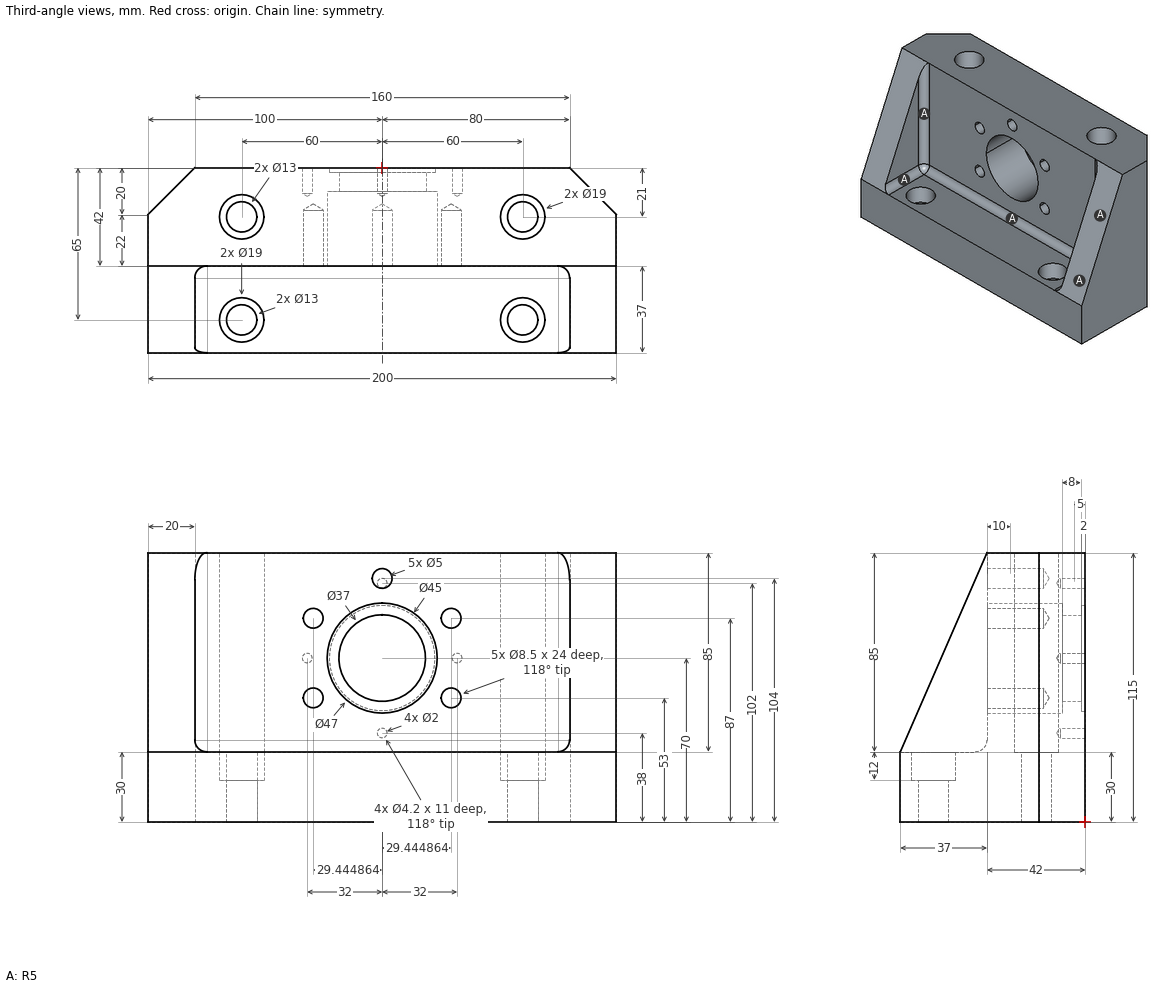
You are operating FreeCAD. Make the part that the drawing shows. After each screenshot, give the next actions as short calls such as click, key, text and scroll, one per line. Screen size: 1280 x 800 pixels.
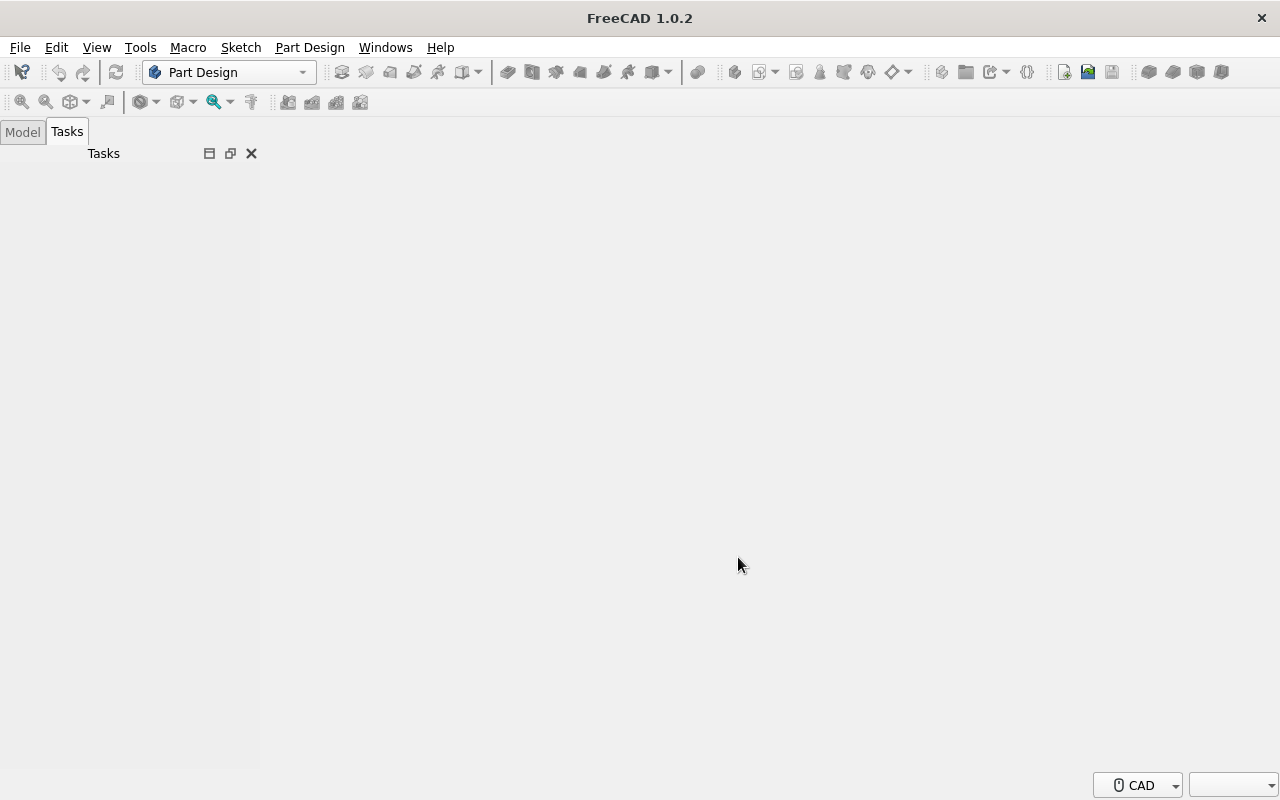
click(1064, 72)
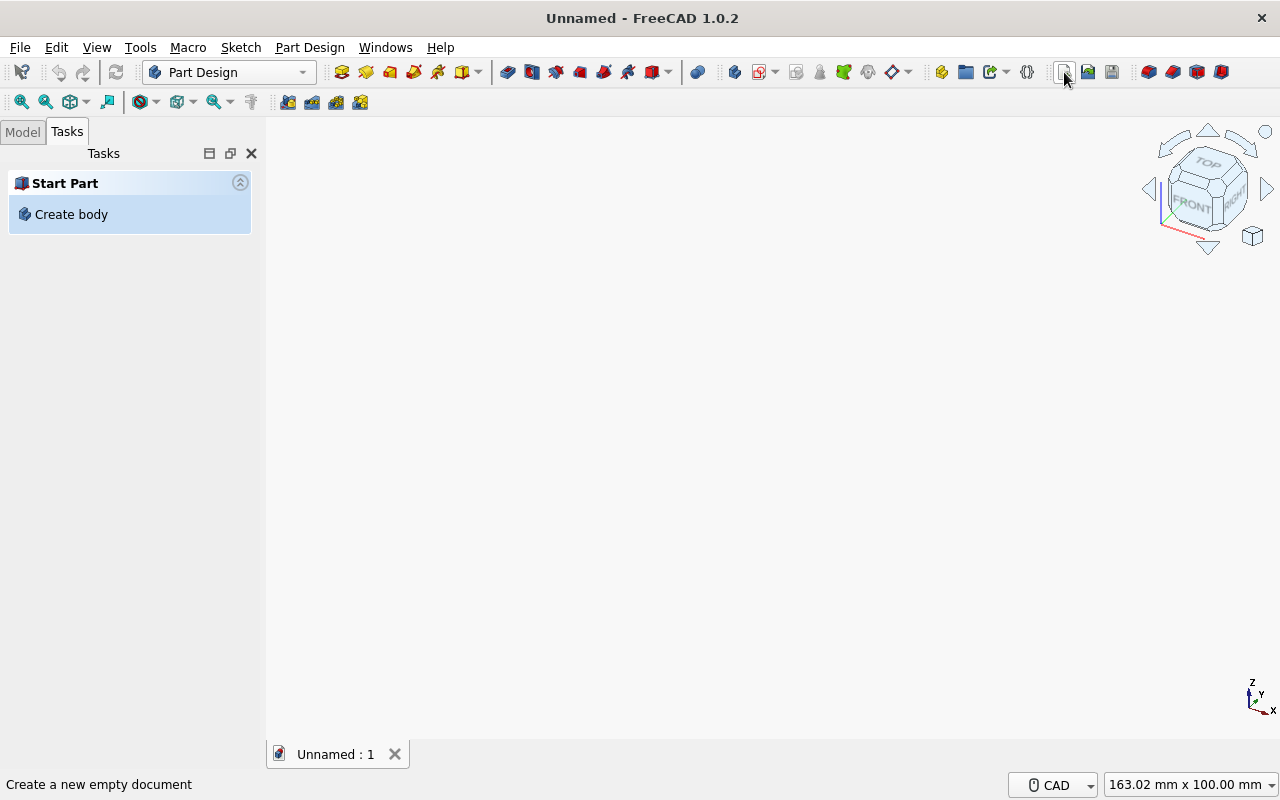
click(760, 72)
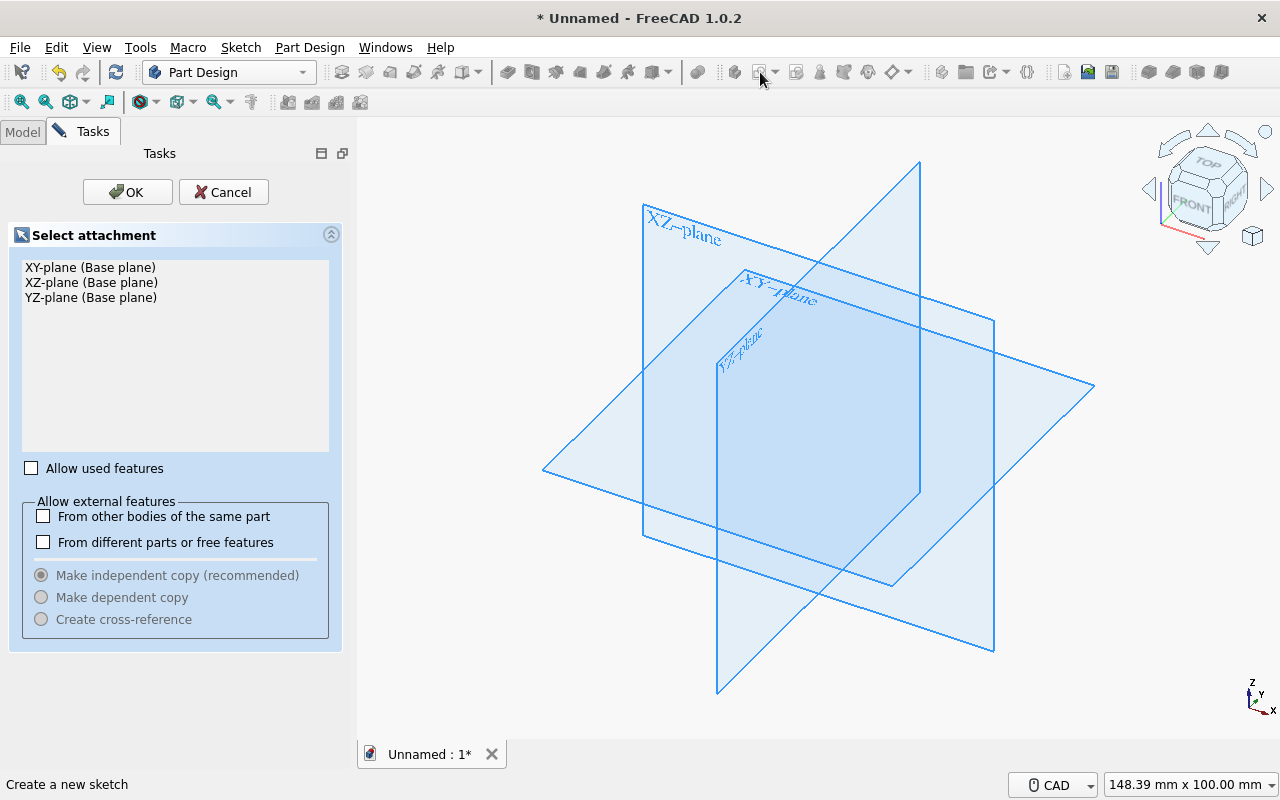
click(82, 268)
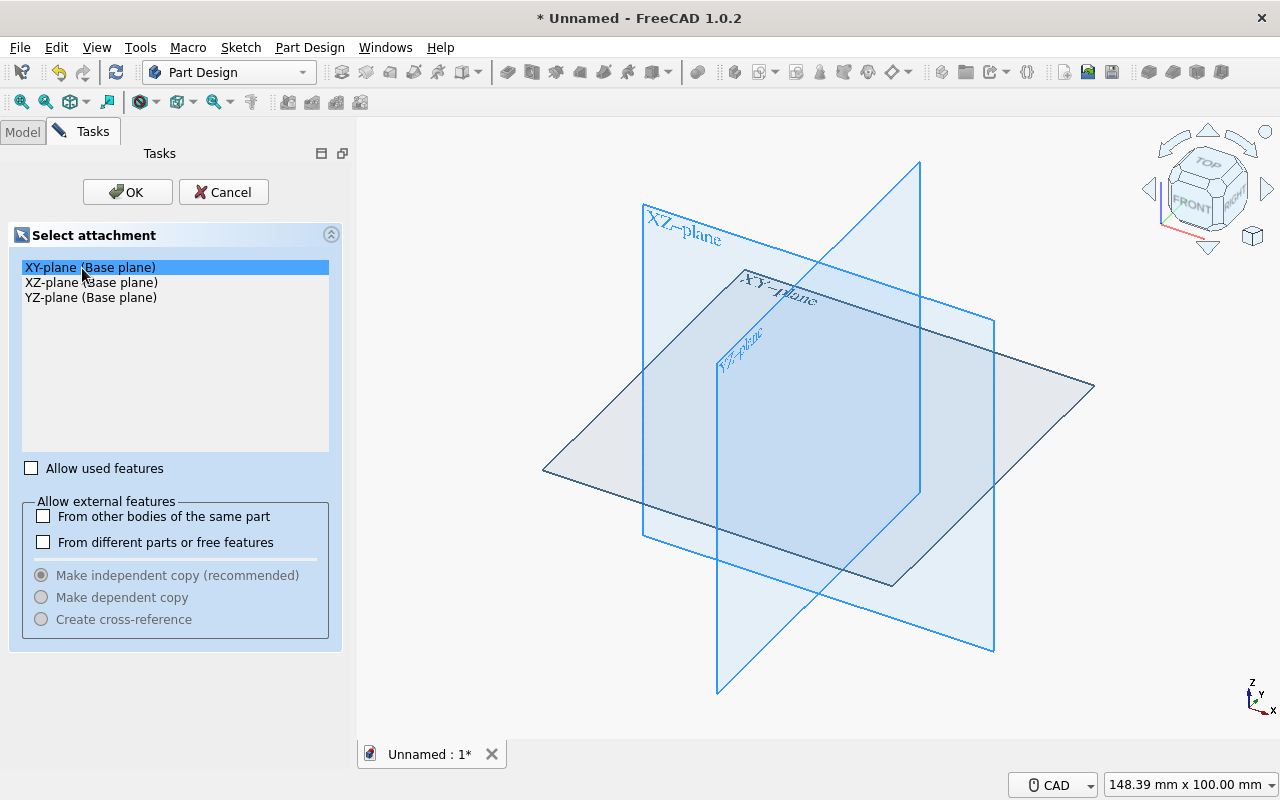
click(128, 192)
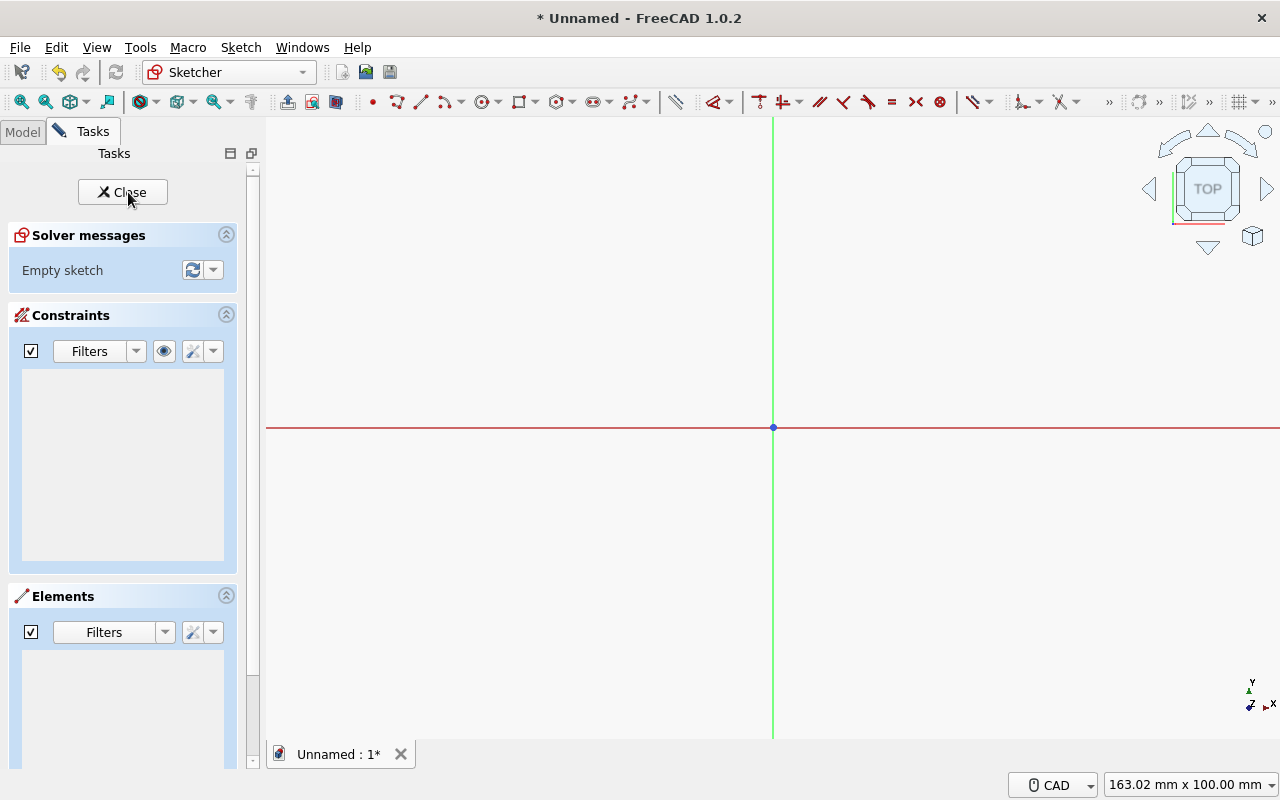
scroll(649, 321, down, 4)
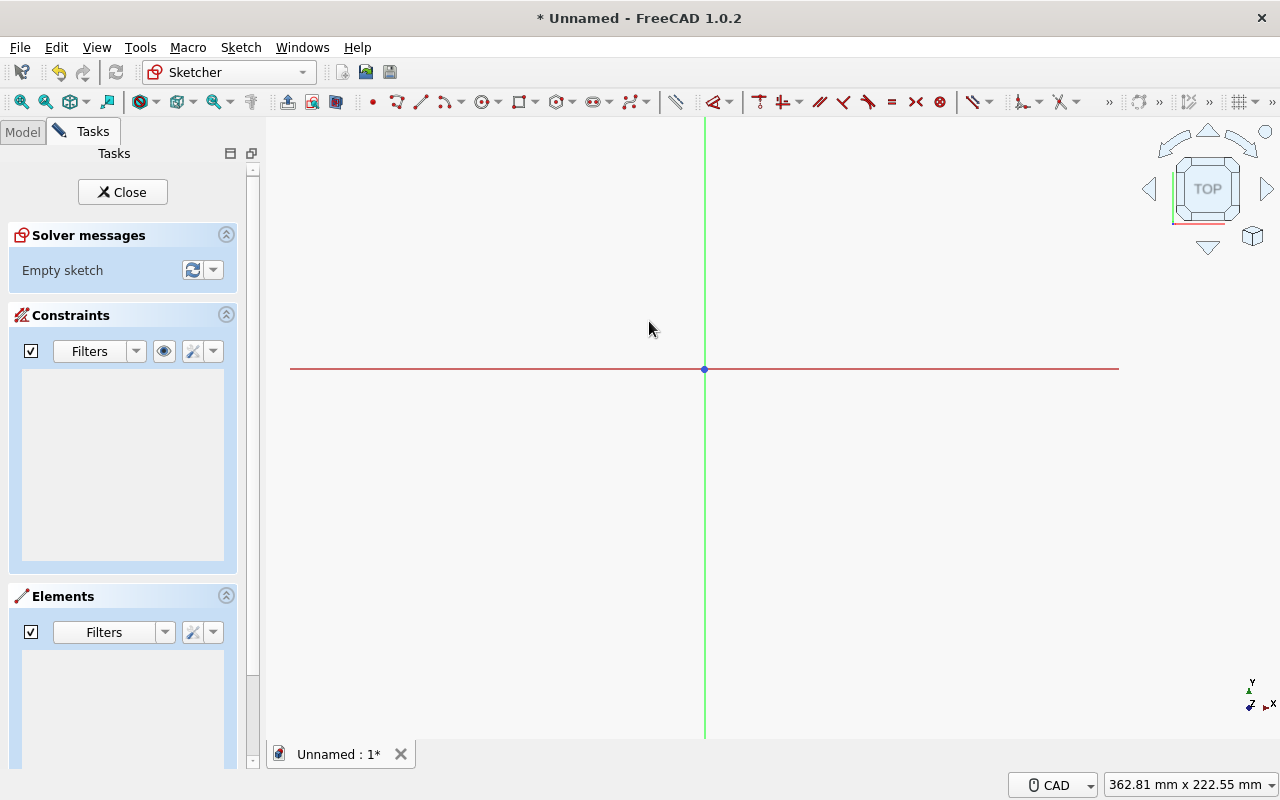
click(398, 102)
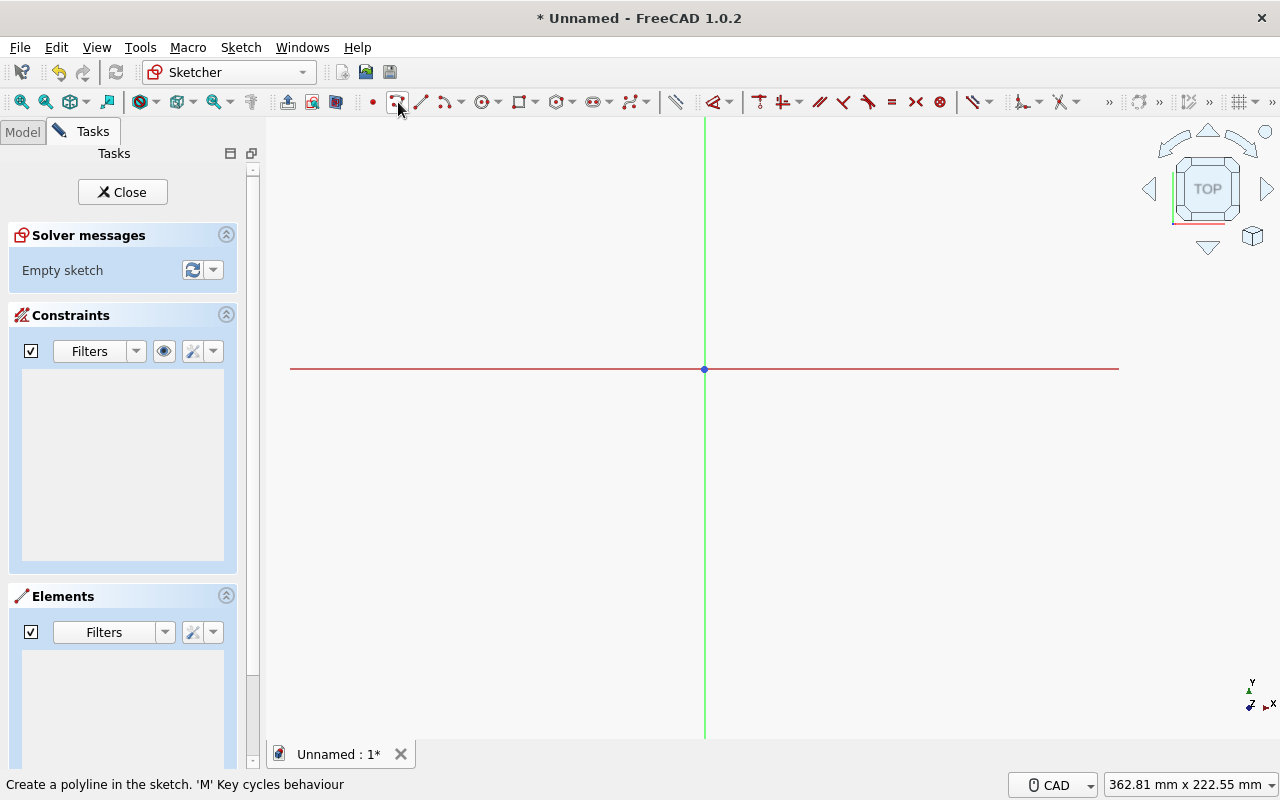
click(929, 369)
click(481, 378)
click(425, 425)
click(425, 487)
click(984, 487)
click(984, 425)
click(929, 369)
key(Escape)
key(Escape)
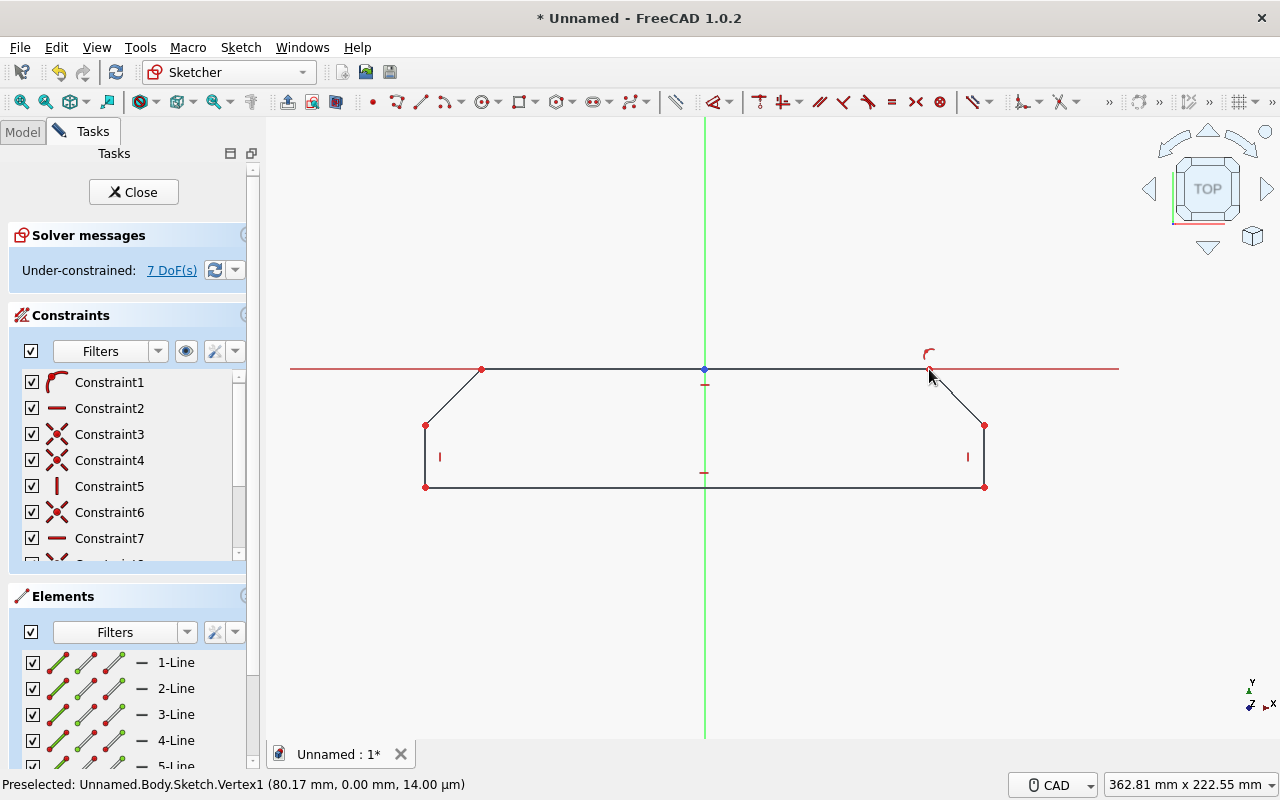
click(425, 426)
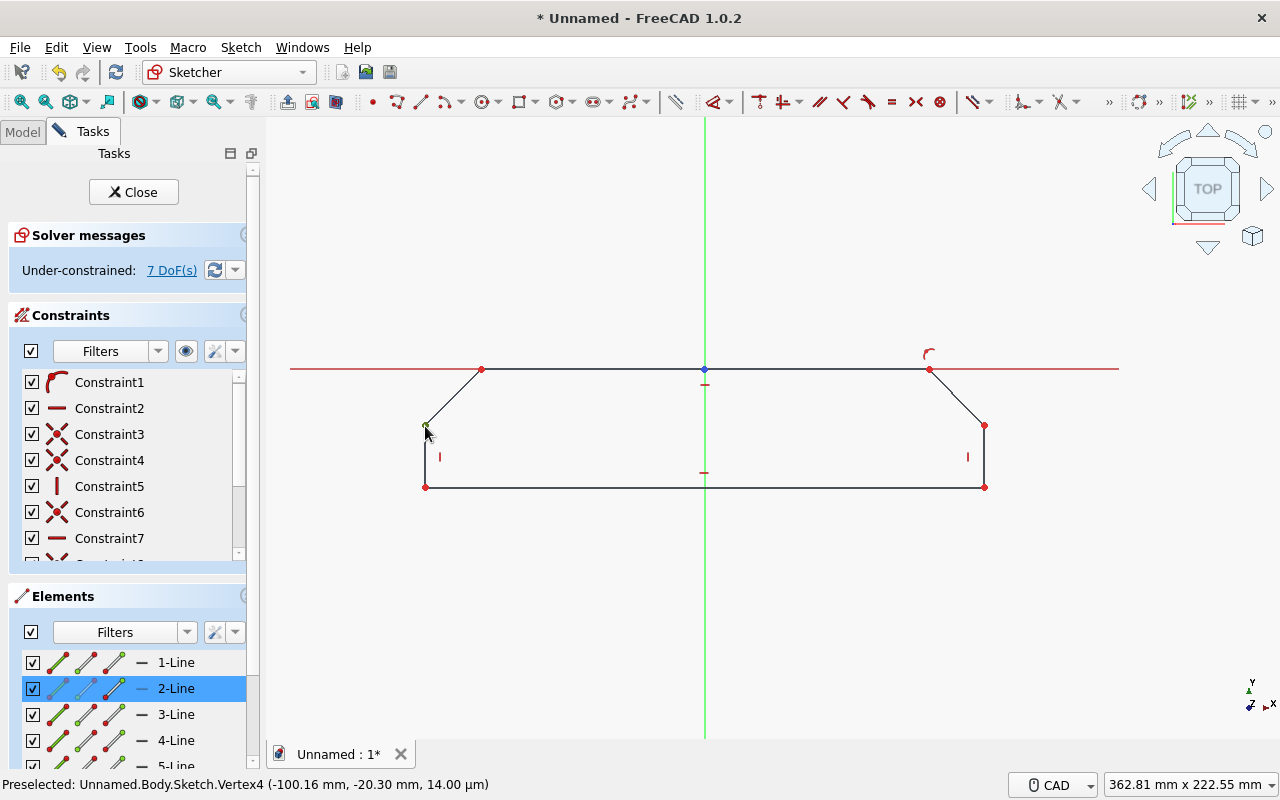
click(984, 426)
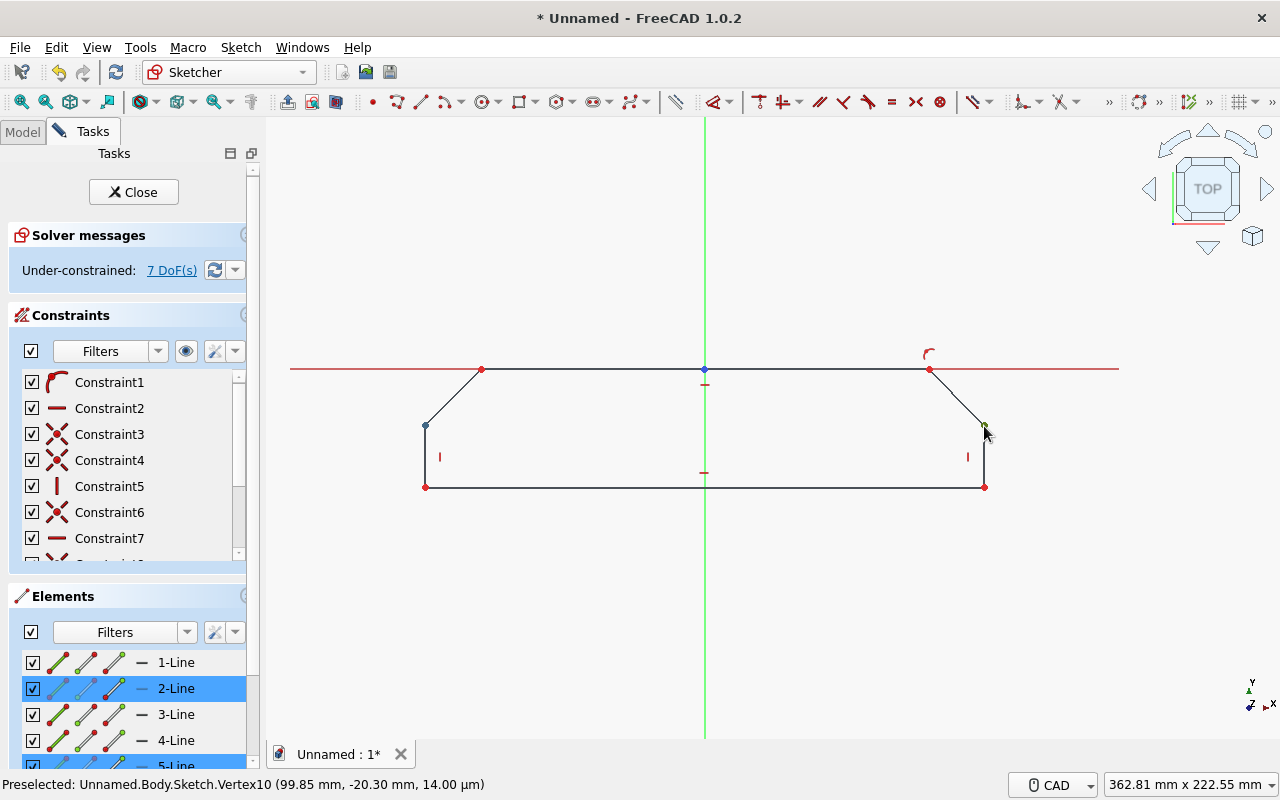
click(705, 671)